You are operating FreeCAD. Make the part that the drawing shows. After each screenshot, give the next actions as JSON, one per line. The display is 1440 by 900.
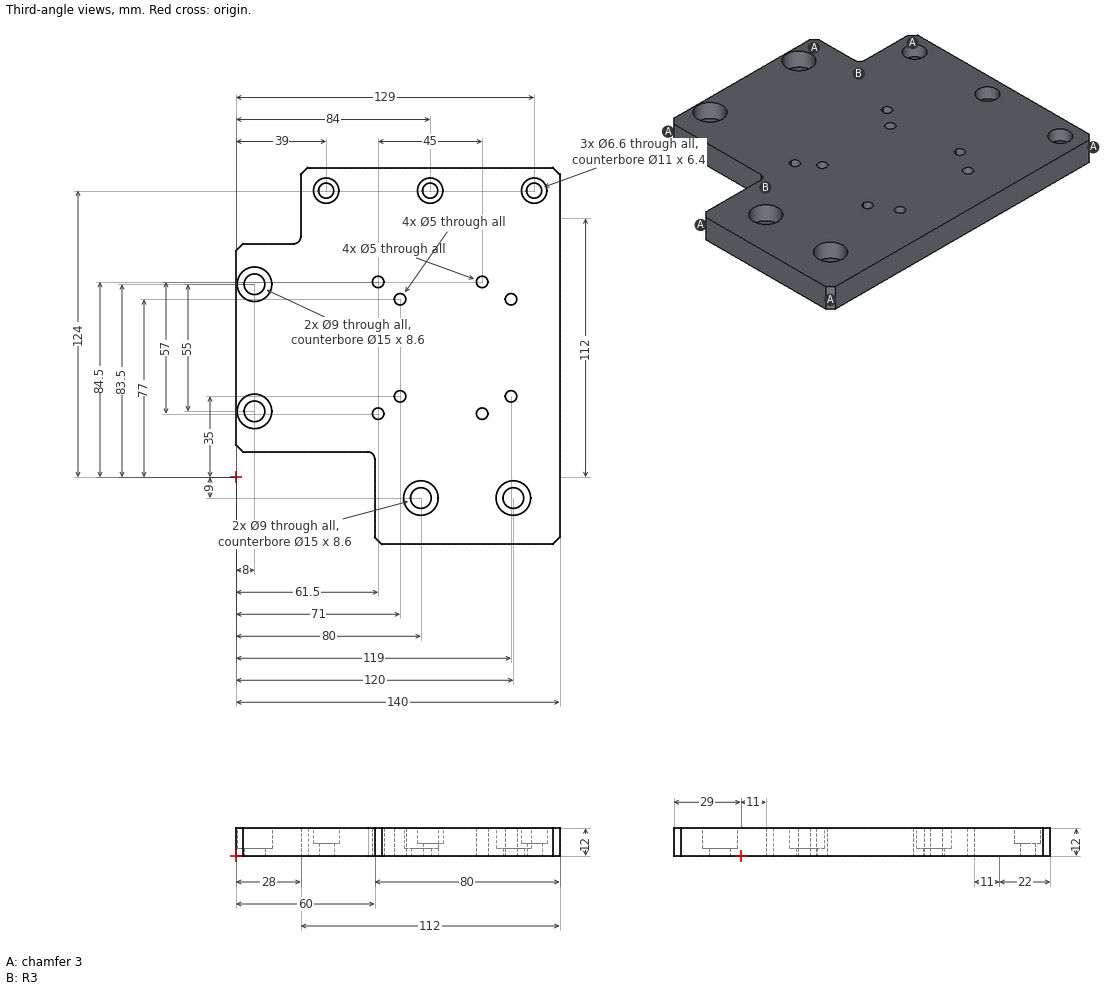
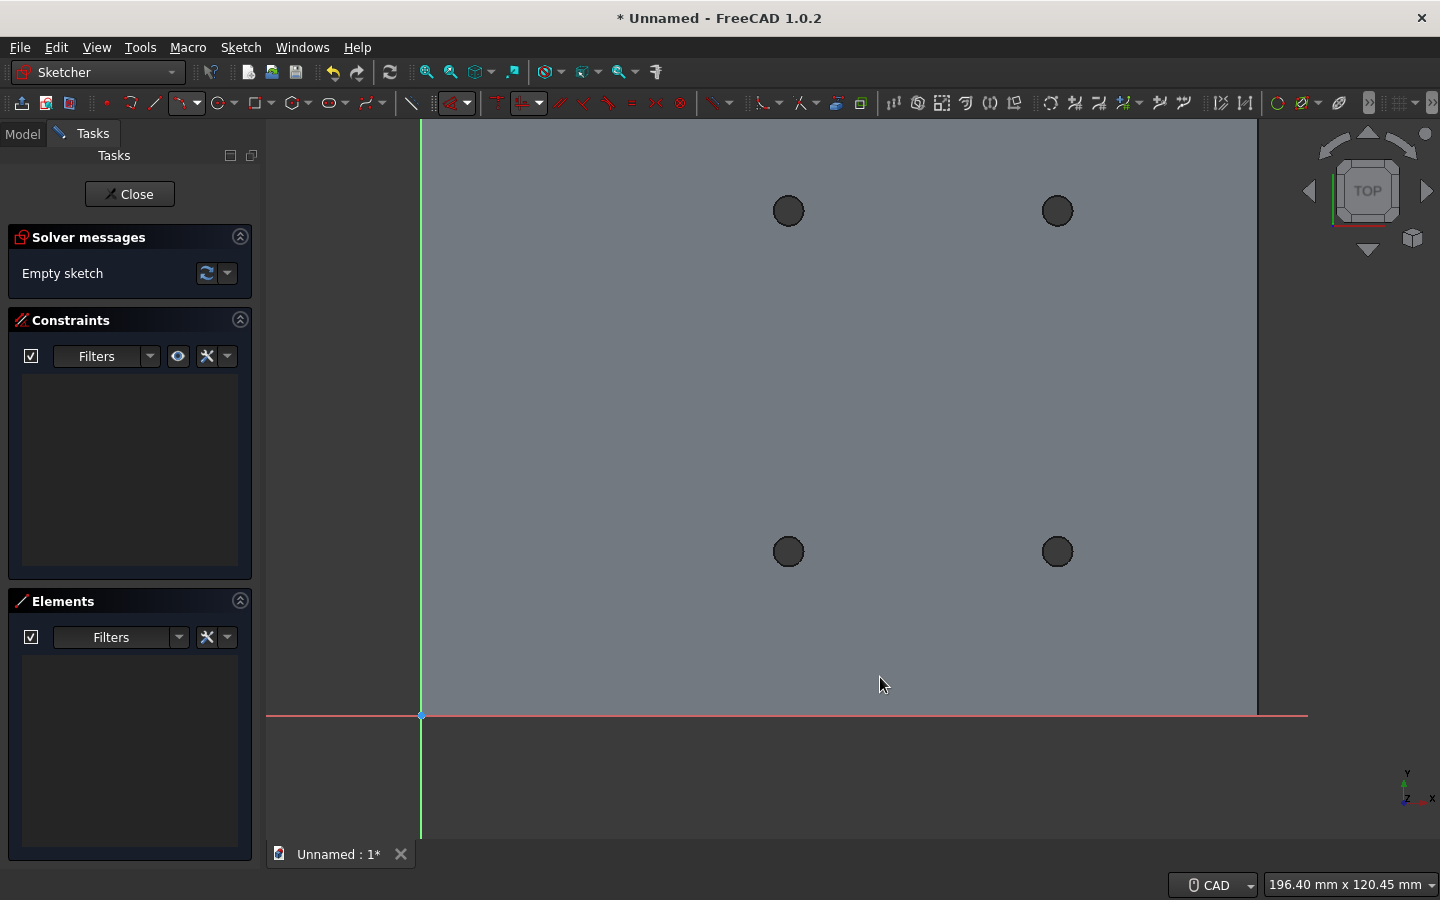
{"action": "left_click", "coordinate": [218, 104]}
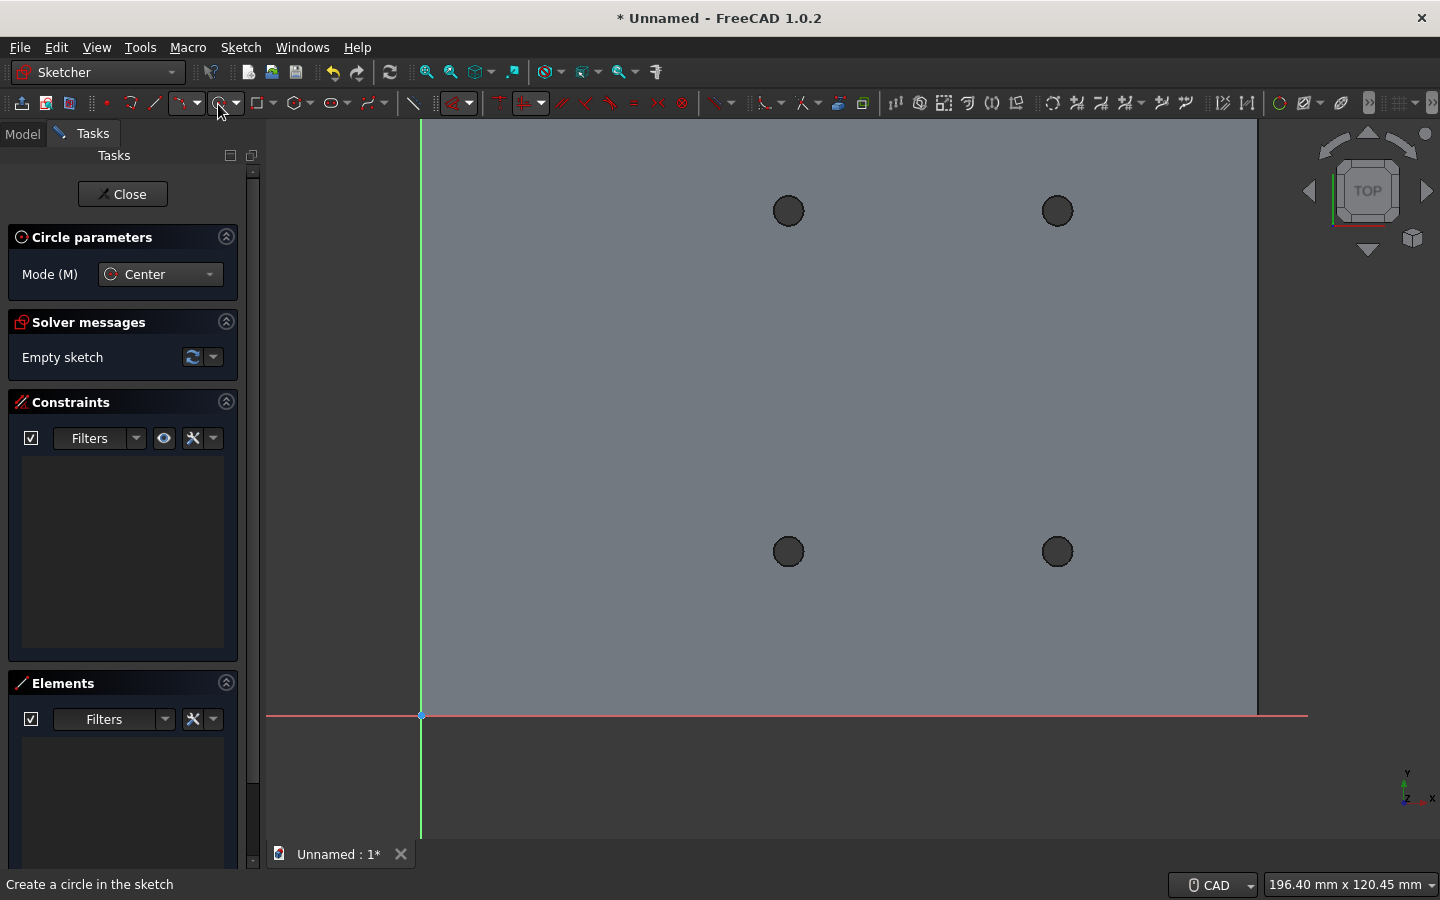
{"action": "scroll", "coordinate": [845, 256], "scroll_direction": "up", "scroll_amount": 3}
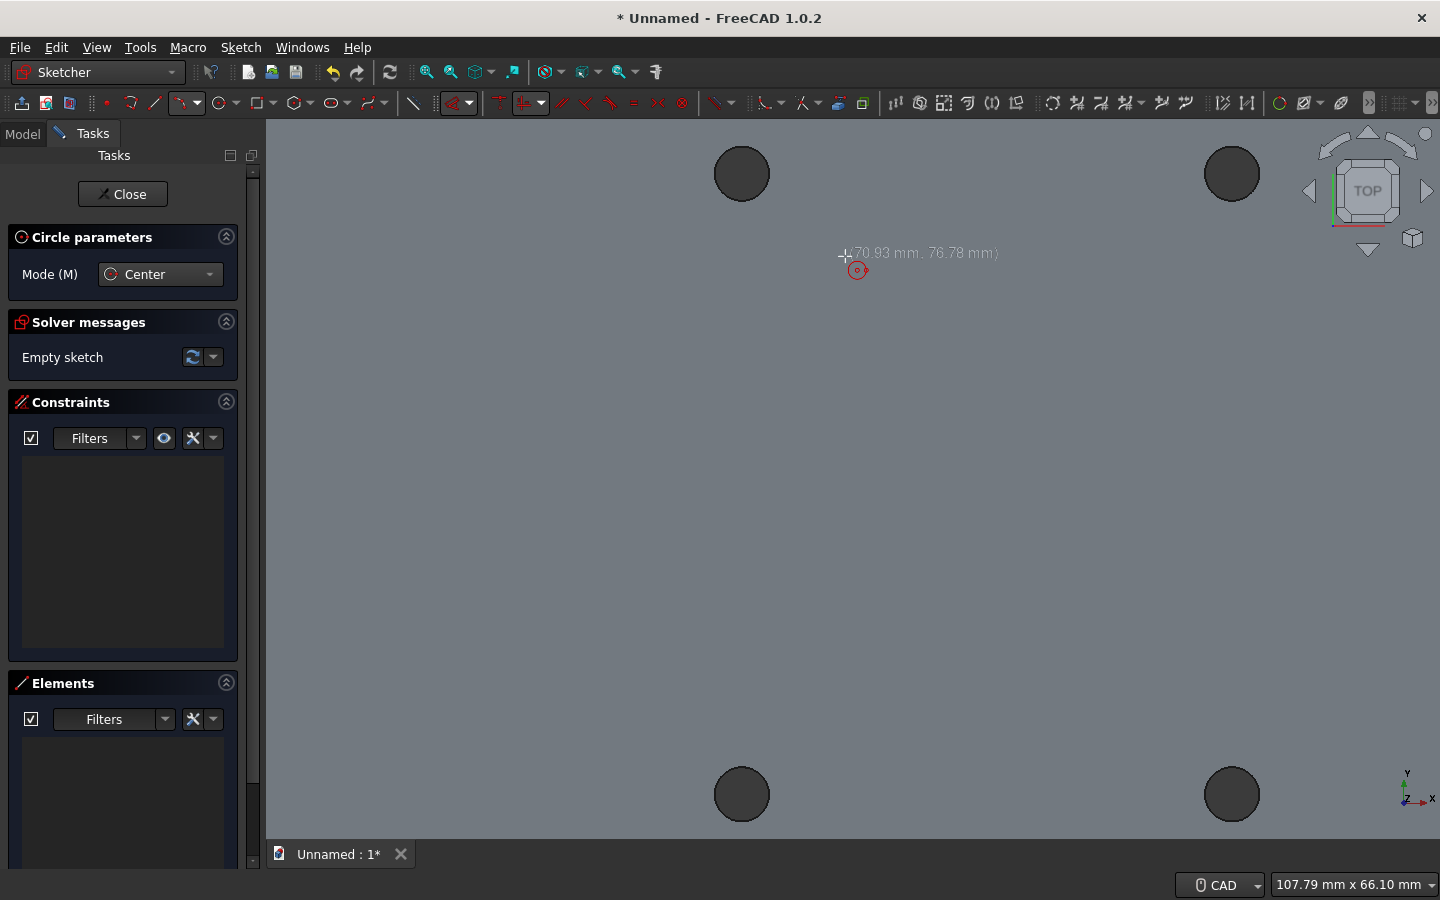
{"action": "left_click", "coordinate": [845, 255]}
{"action": "mouse_move", "coordinate": [865, 236]}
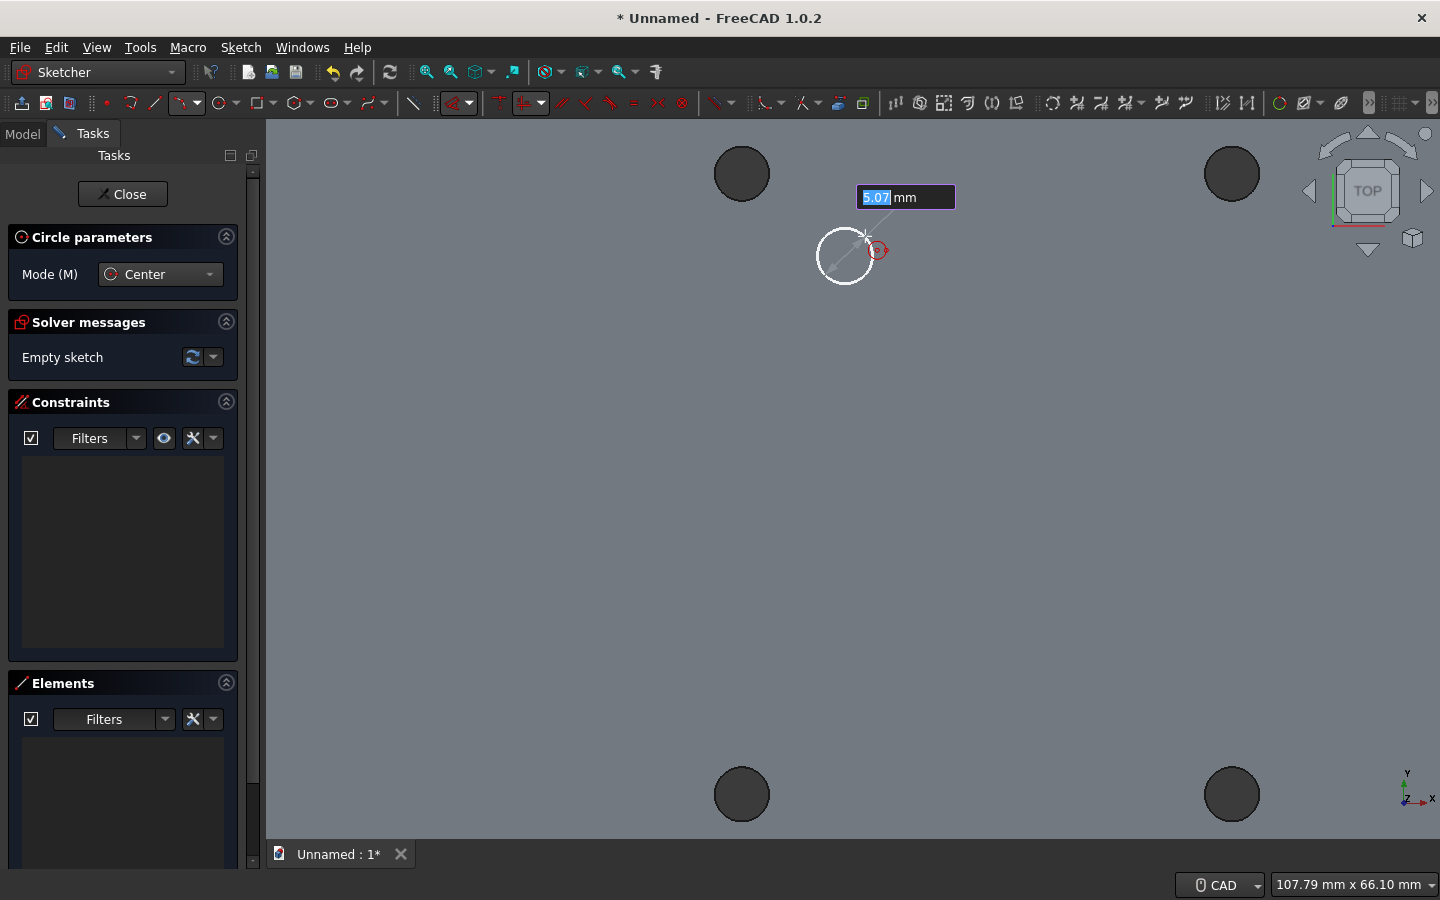
{"action": "type", "text": "5"}
{"action": "key", "text": "Return"}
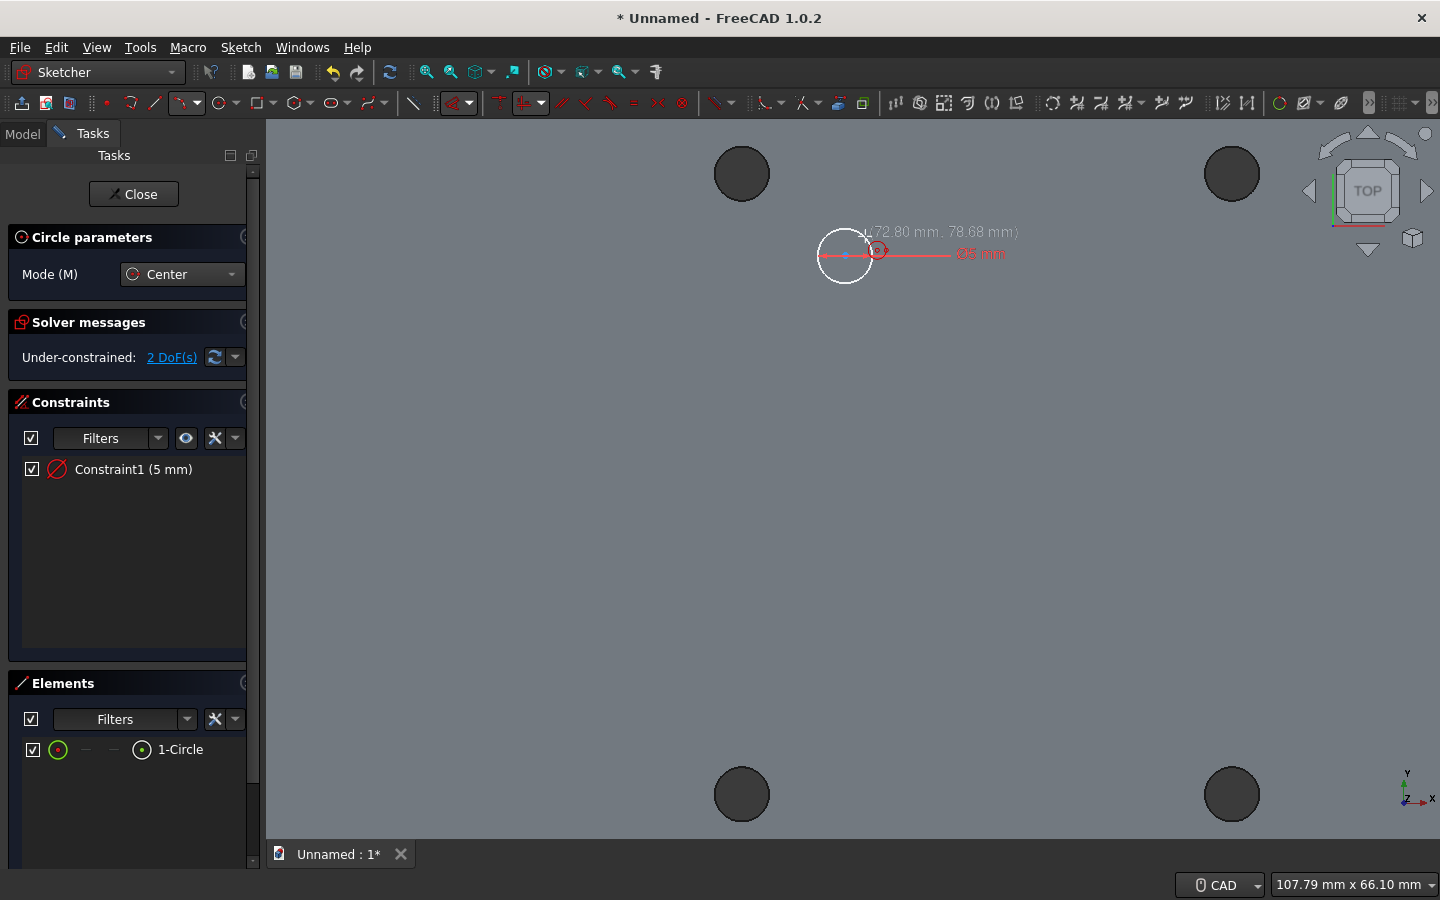
{"action": "left_click", "coordinate": [845, 713]}
{"action": "mouse_move", "coordinate": [865, 694]}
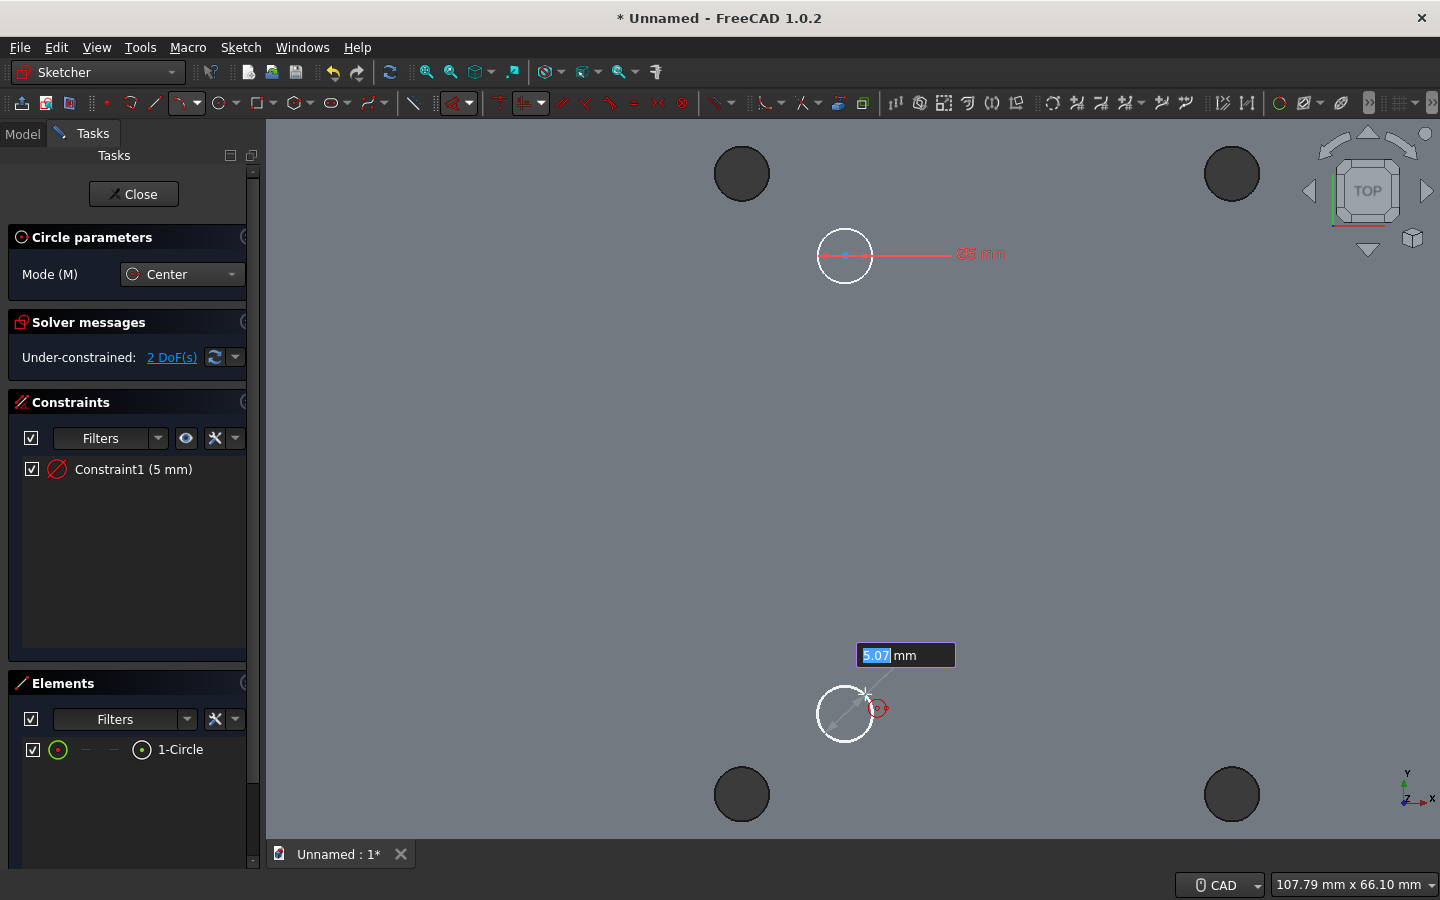
{"action": "type", "text": "5"}
{"action": "key", "text": "Return"}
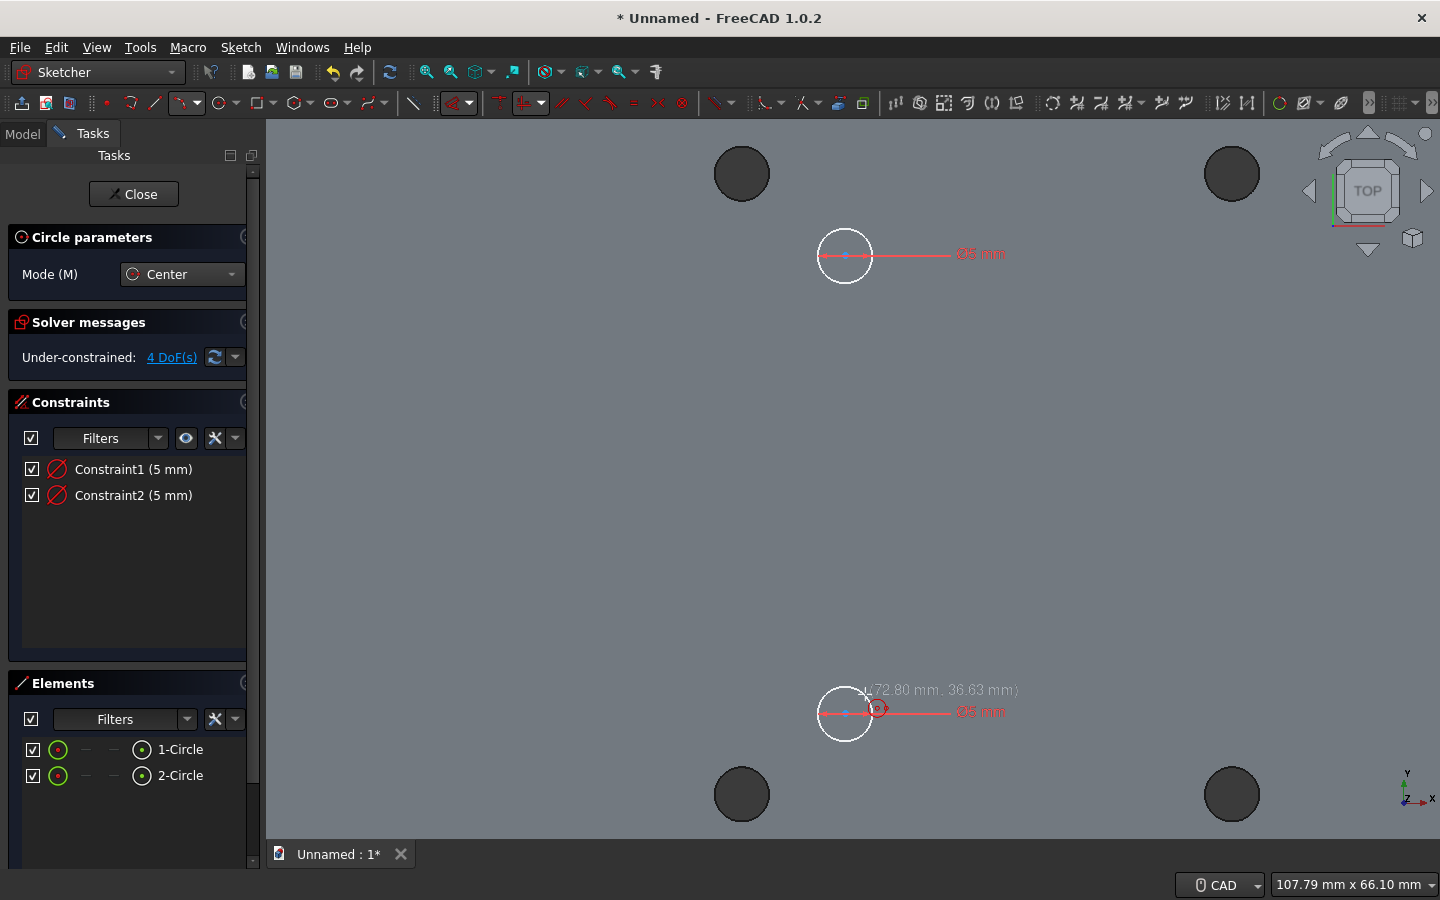
{"action": "scroll", "coordinate": [846, 258], "scroll_direction": "down", "scroll_amount": 3}